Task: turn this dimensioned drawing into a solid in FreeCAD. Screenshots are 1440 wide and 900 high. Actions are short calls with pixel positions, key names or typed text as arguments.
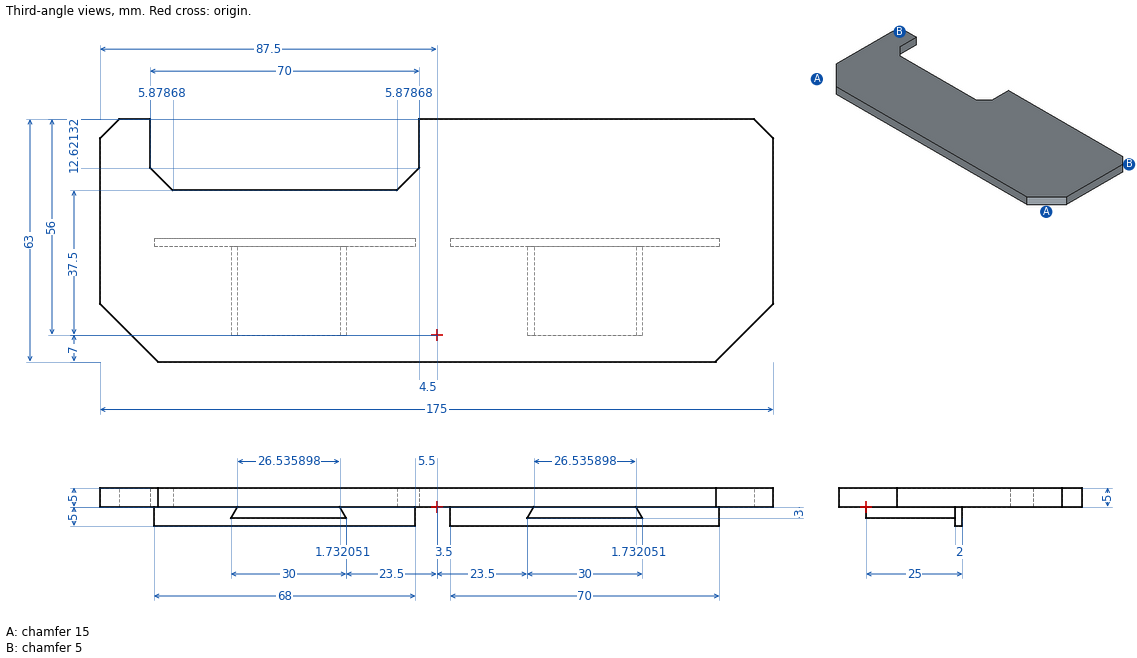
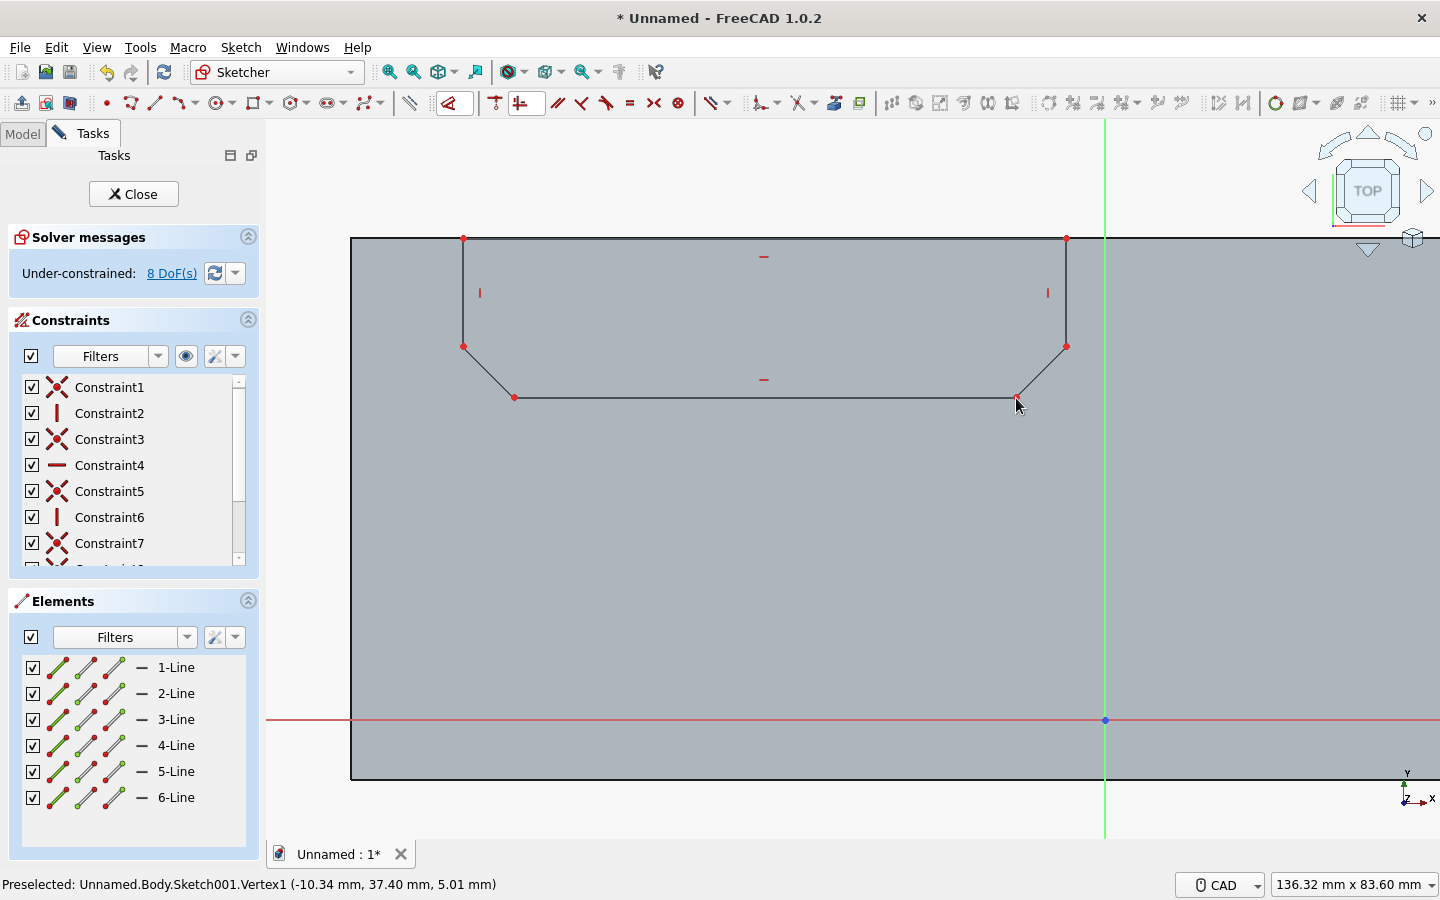
click(885, 239)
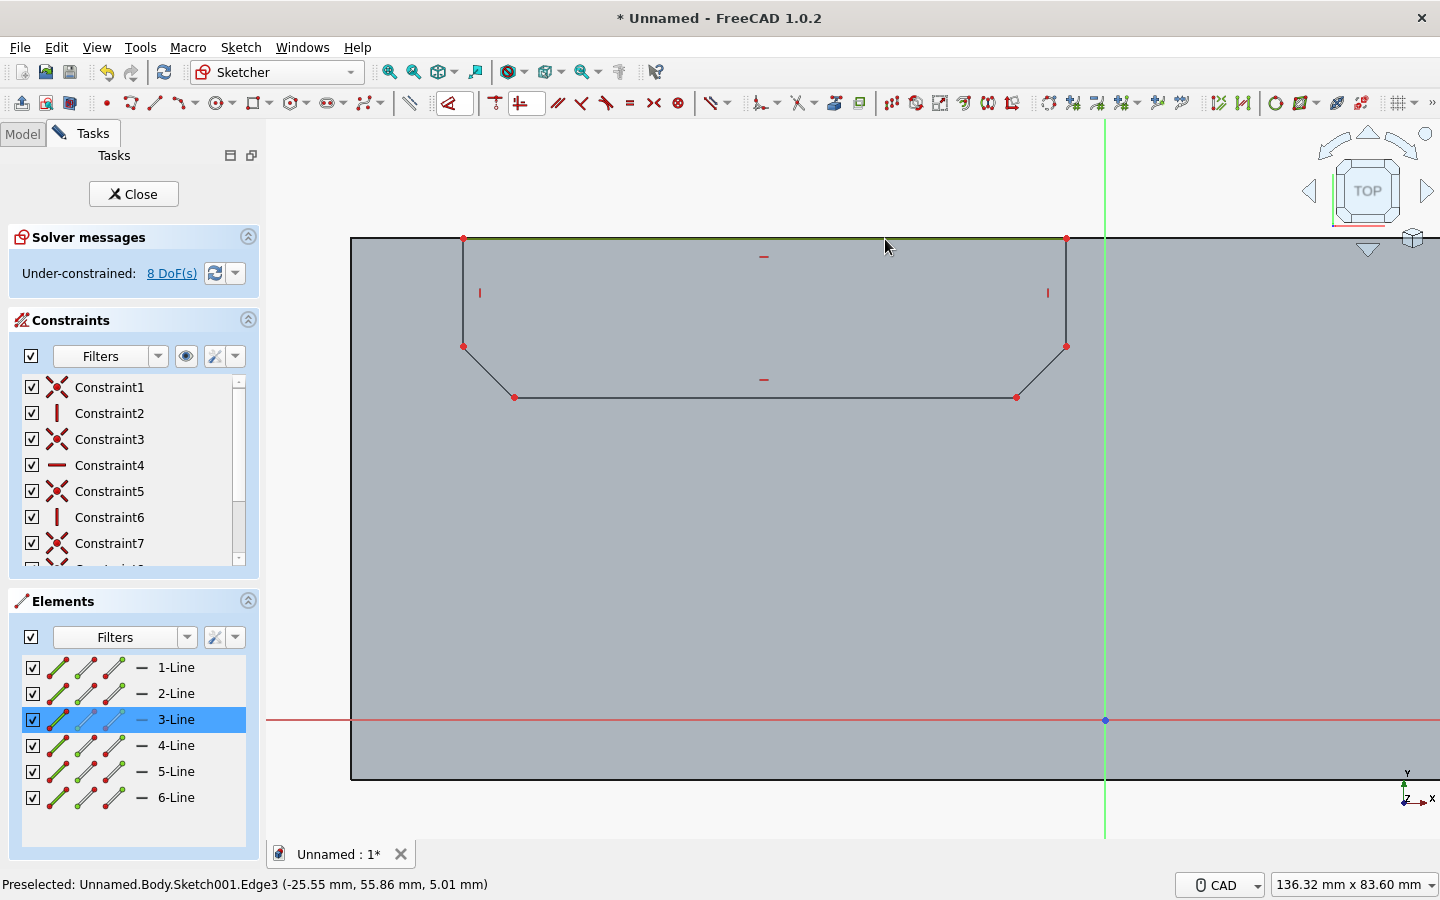
click(468, 104)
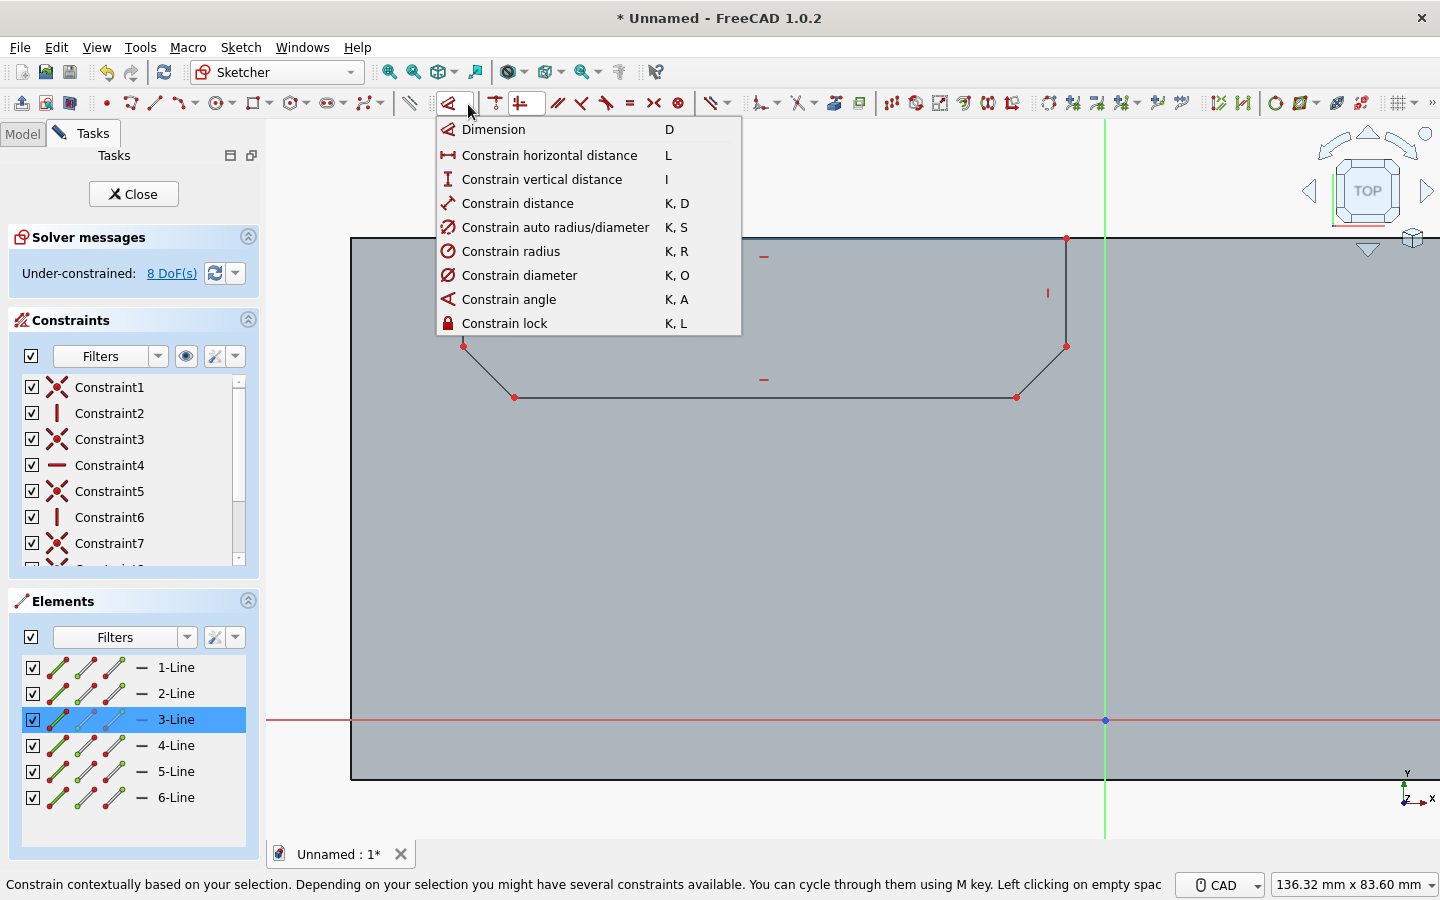
click(589, 155)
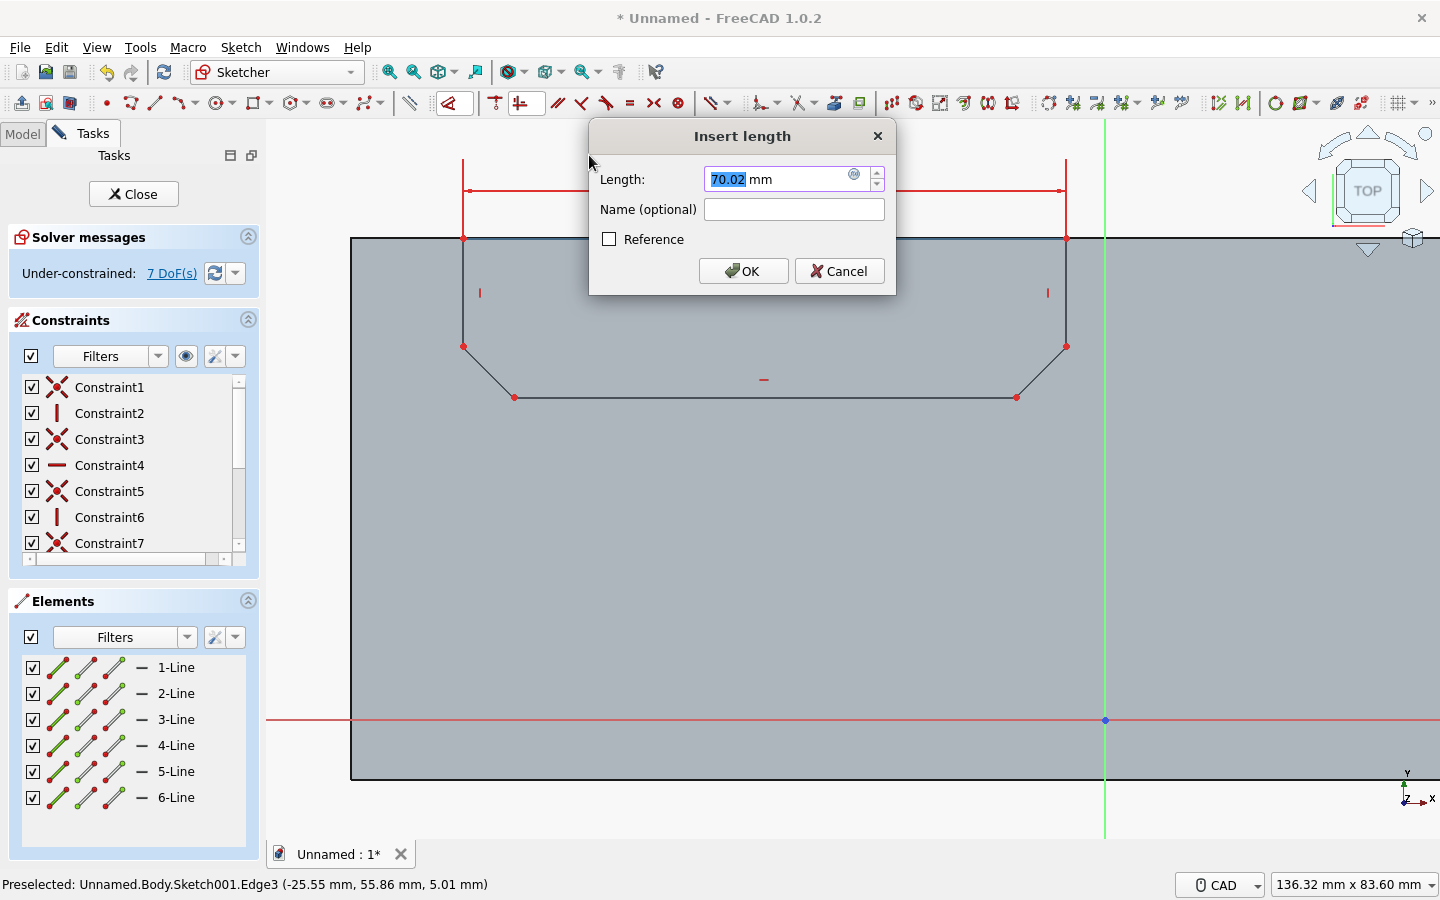
text(70)
key(Return)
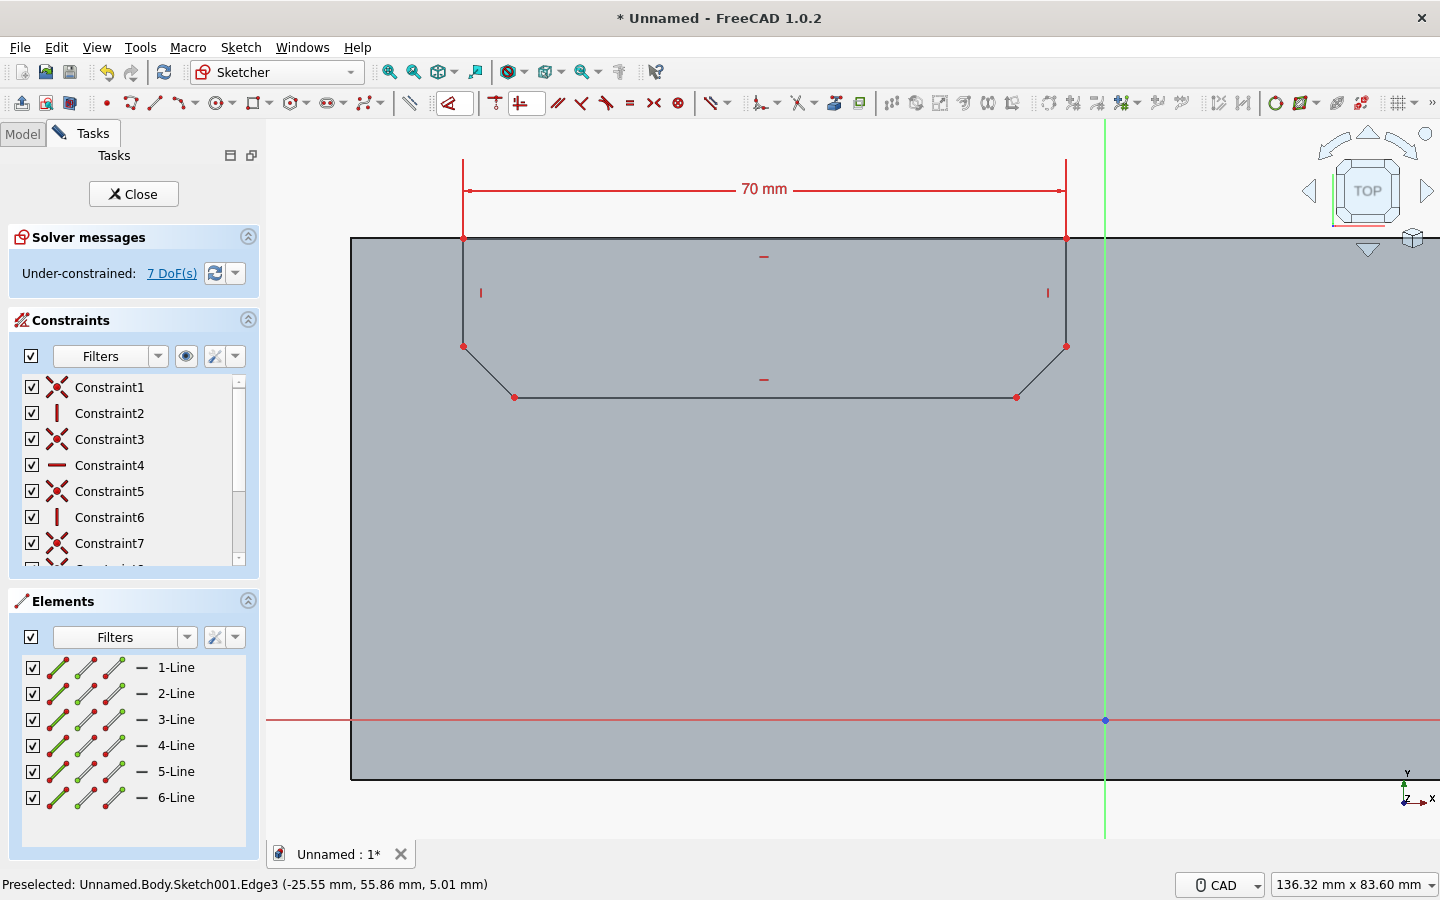
click(1066, 239)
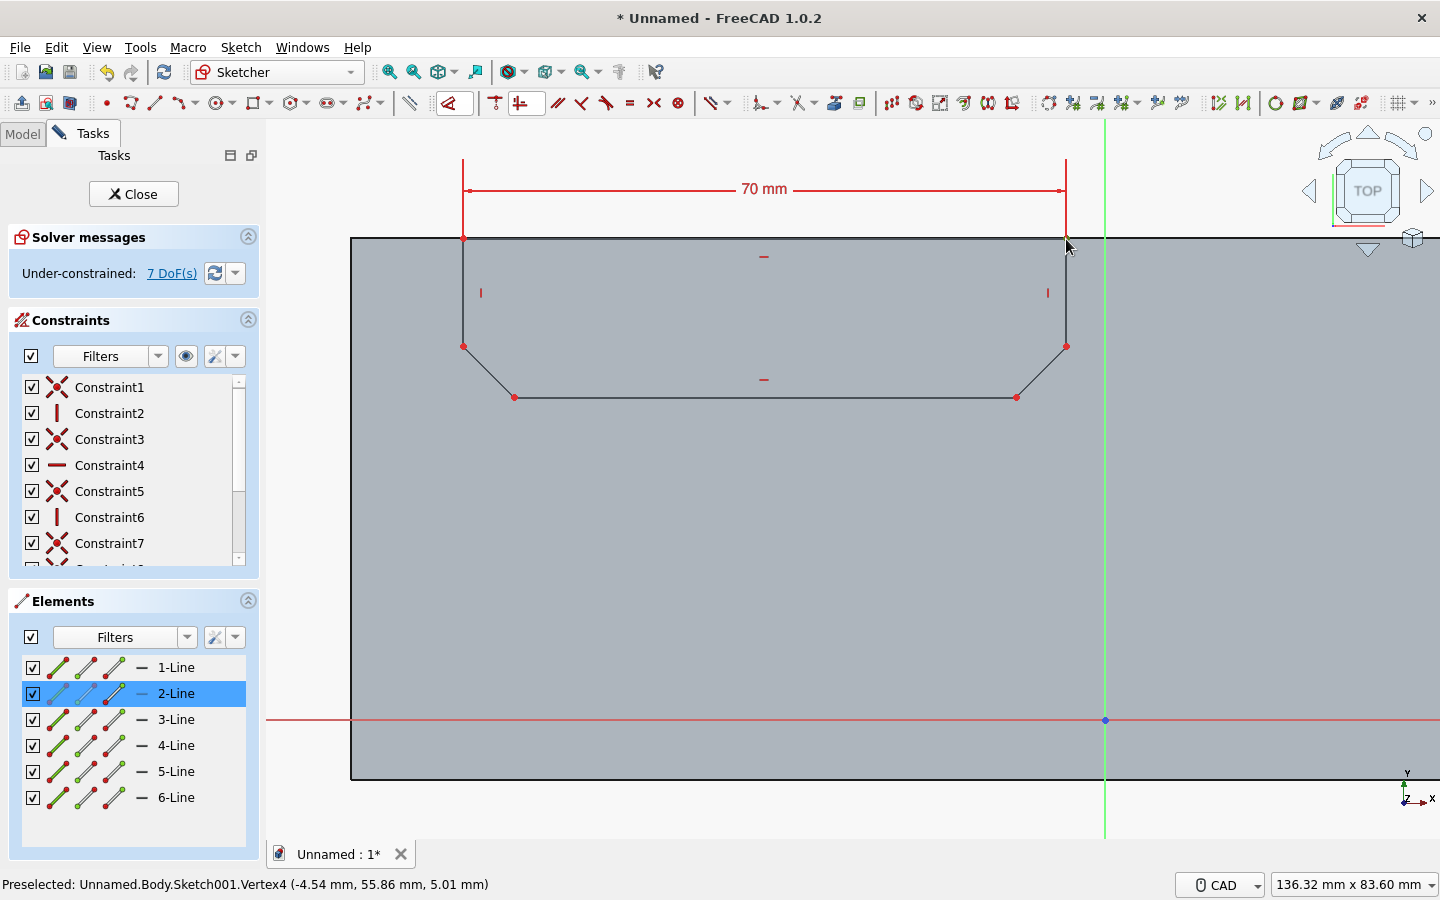
click(468, 104)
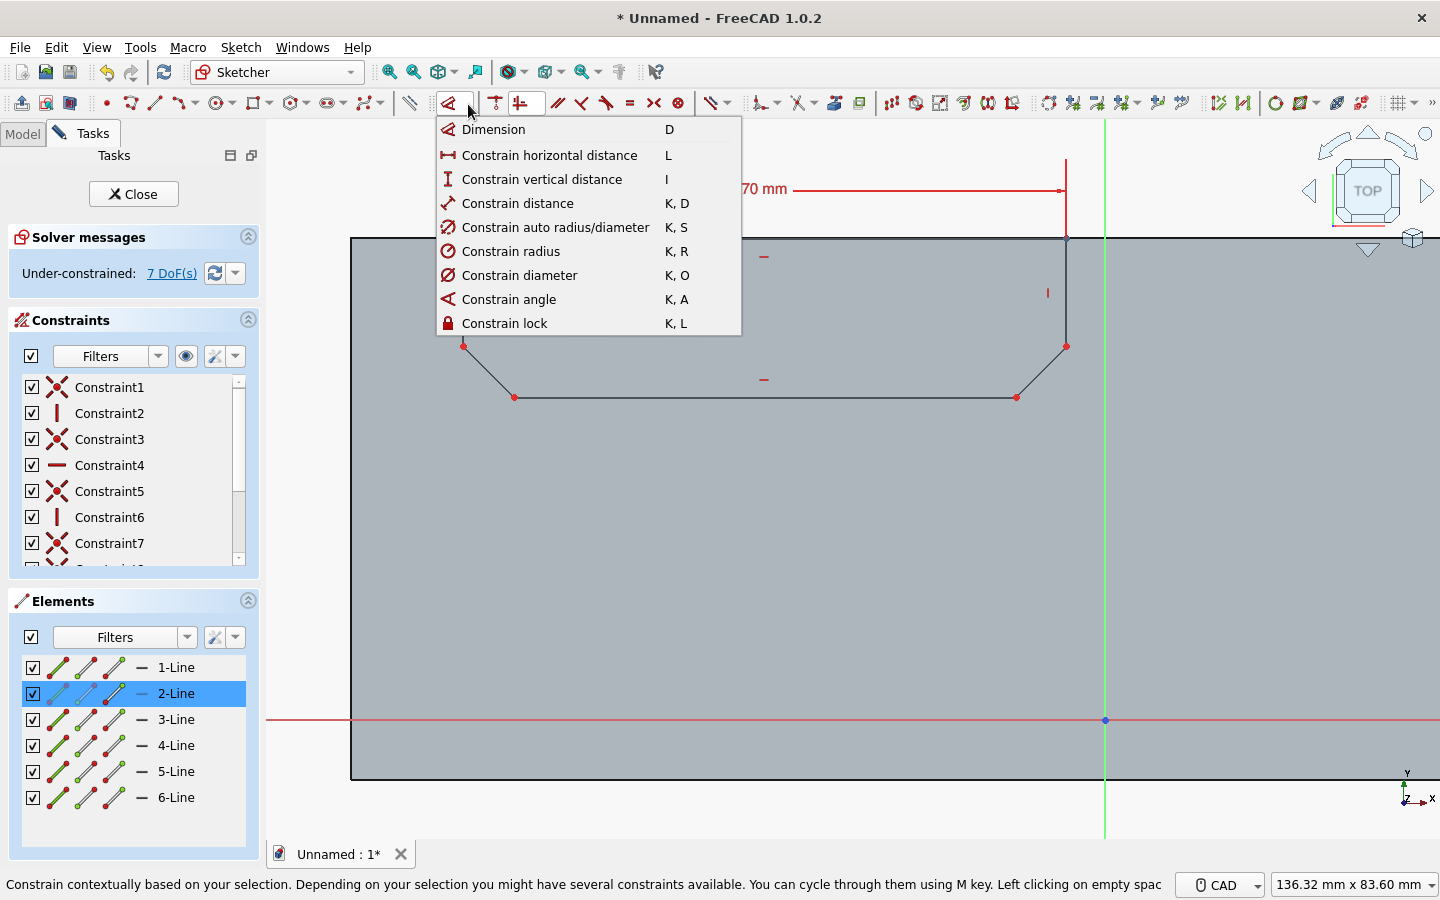
click(589, 179)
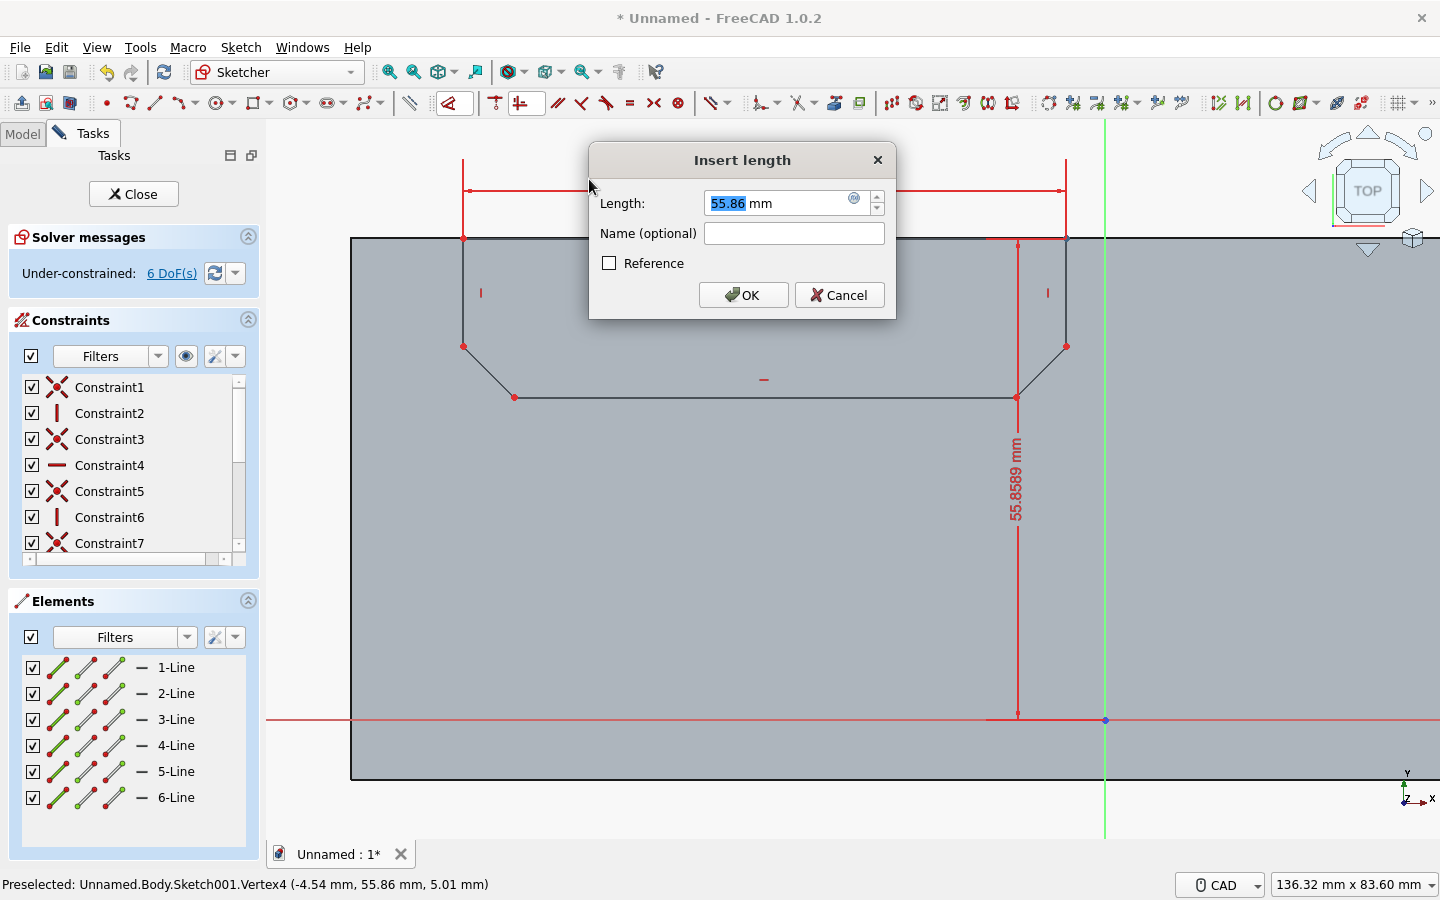
text(56)
key(Return)